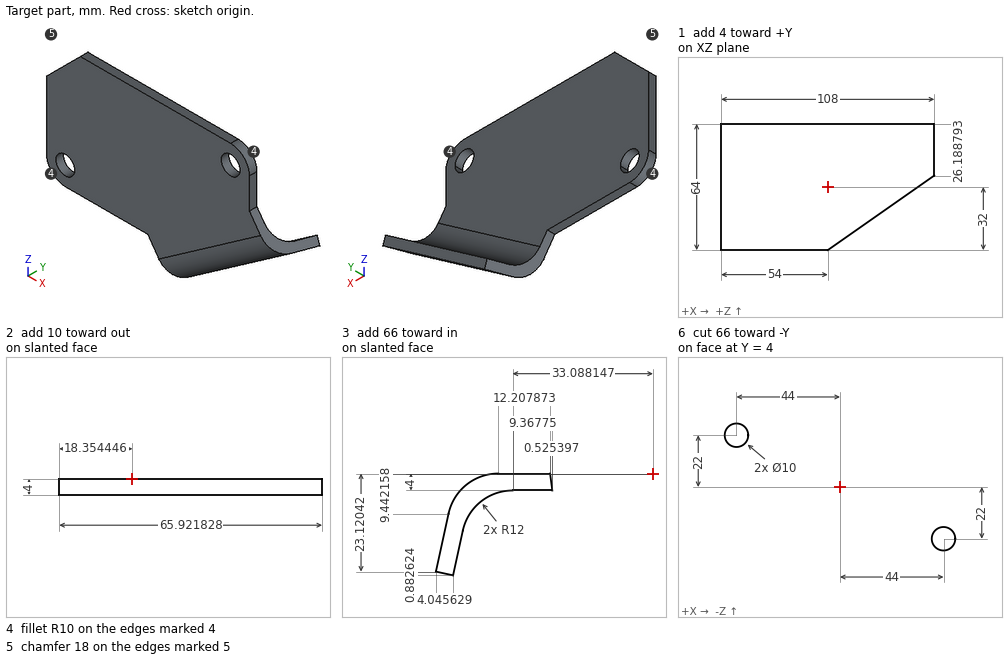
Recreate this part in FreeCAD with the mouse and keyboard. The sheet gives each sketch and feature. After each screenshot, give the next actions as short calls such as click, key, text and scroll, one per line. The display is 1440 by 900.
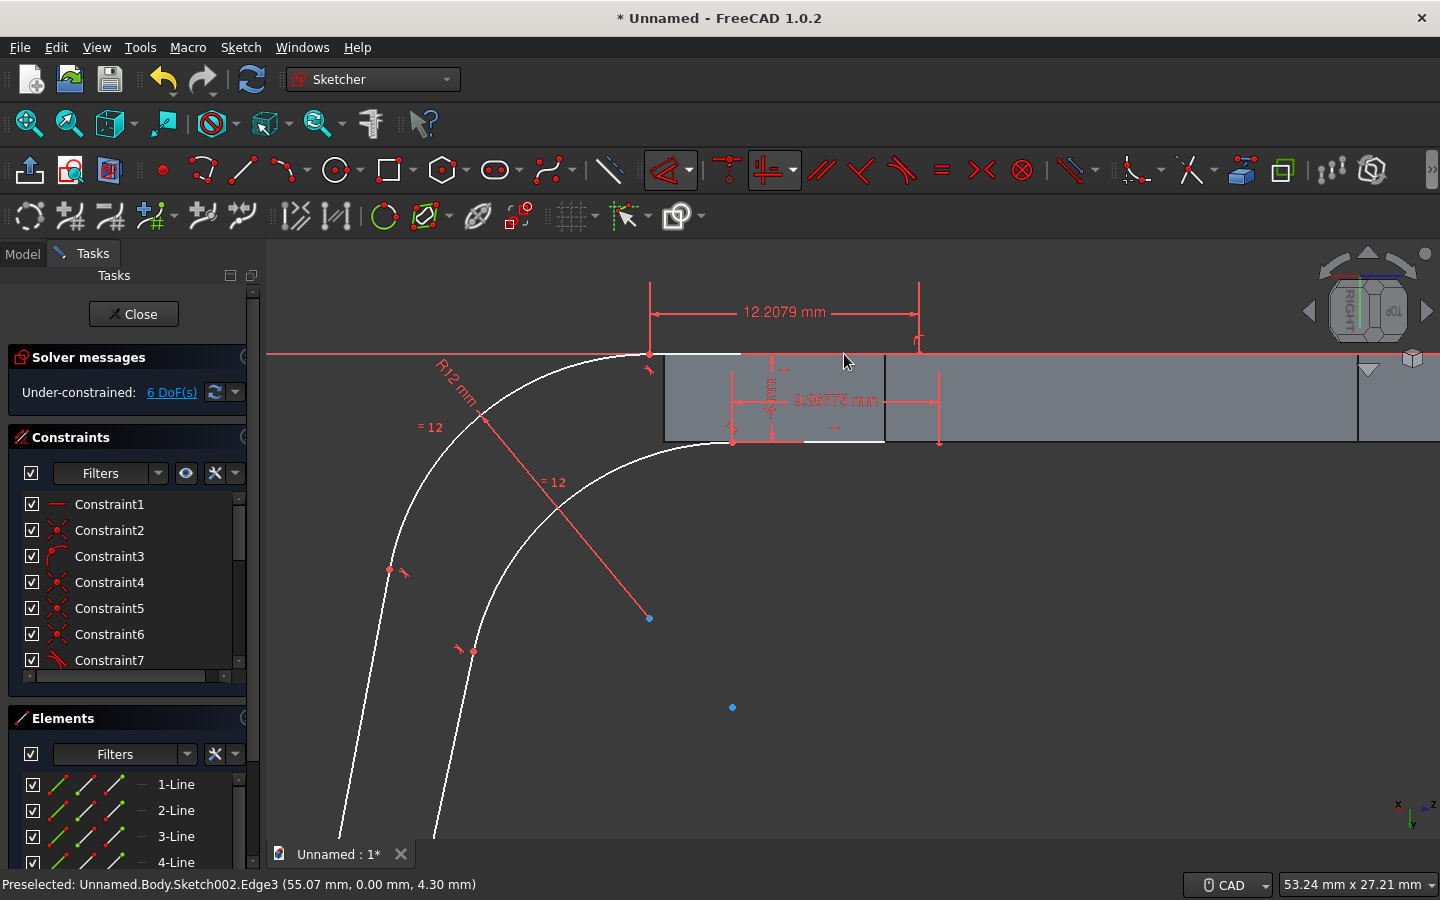
click(390, 570)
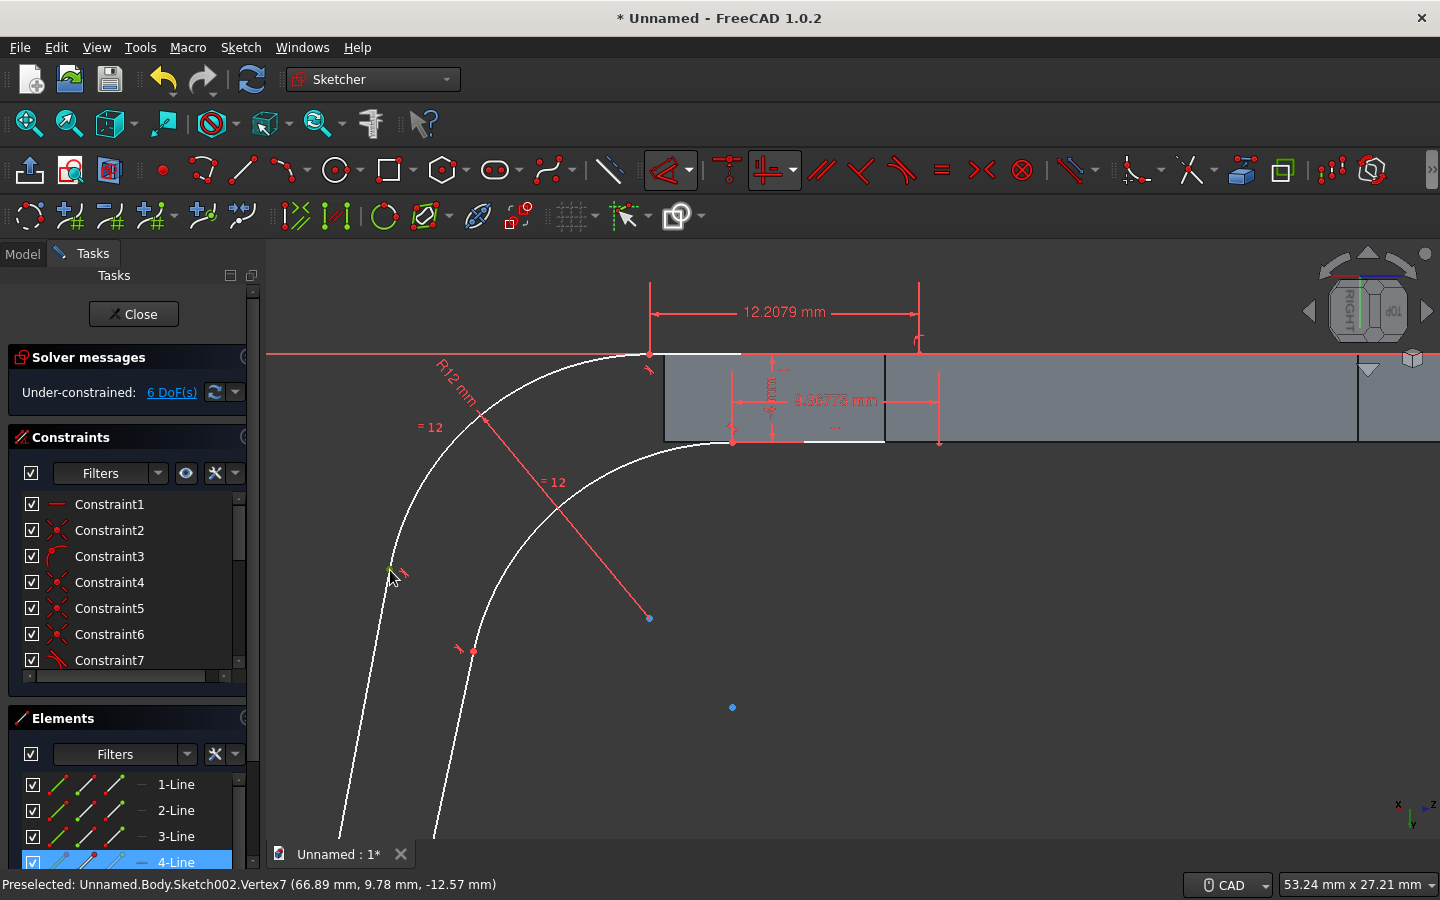
key(i)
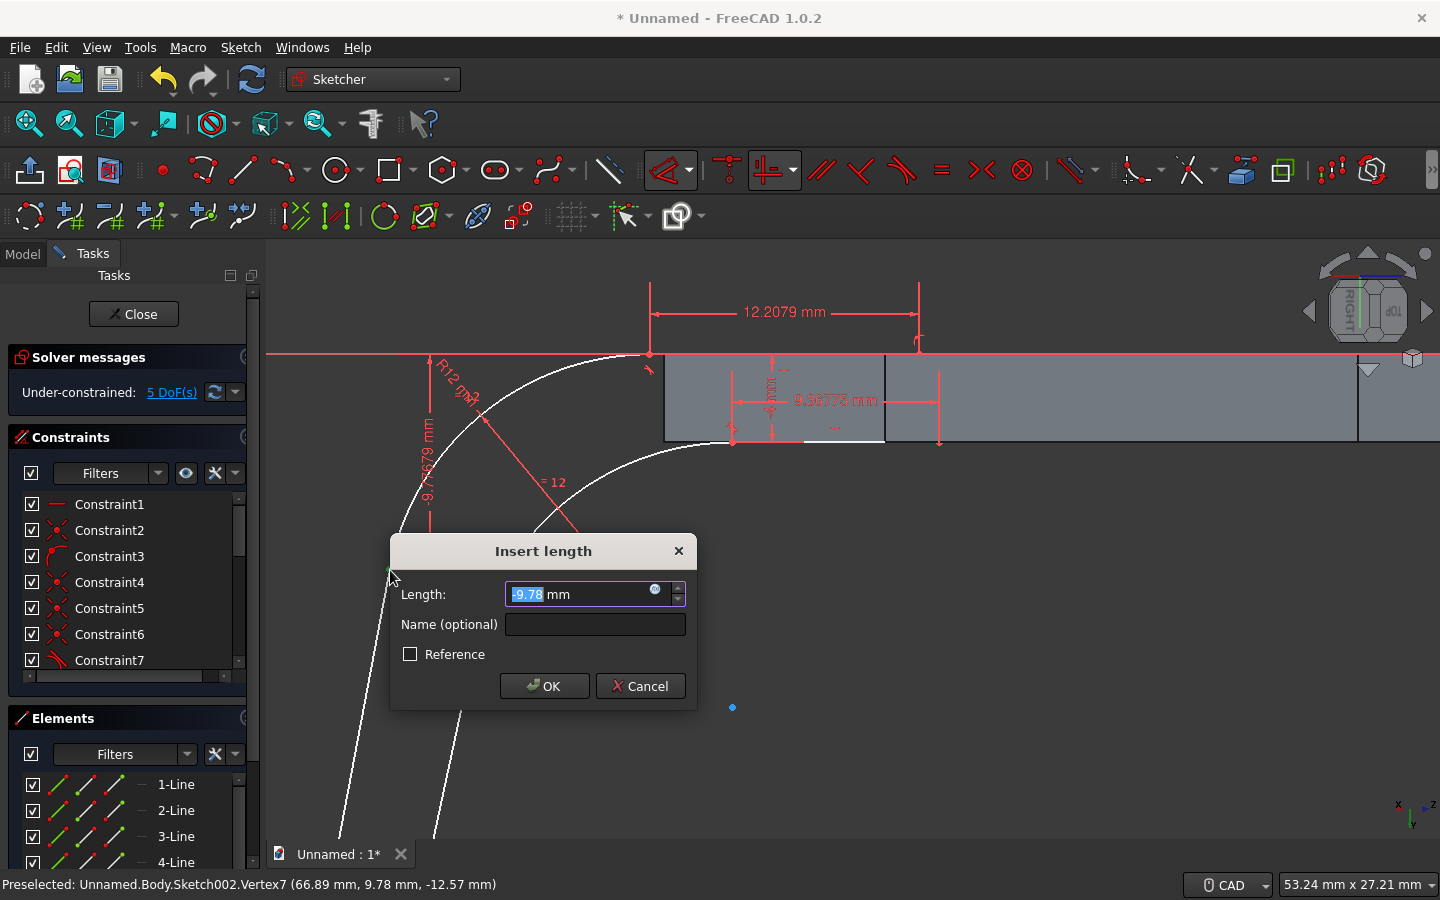
text(-9.442158)
key(Return)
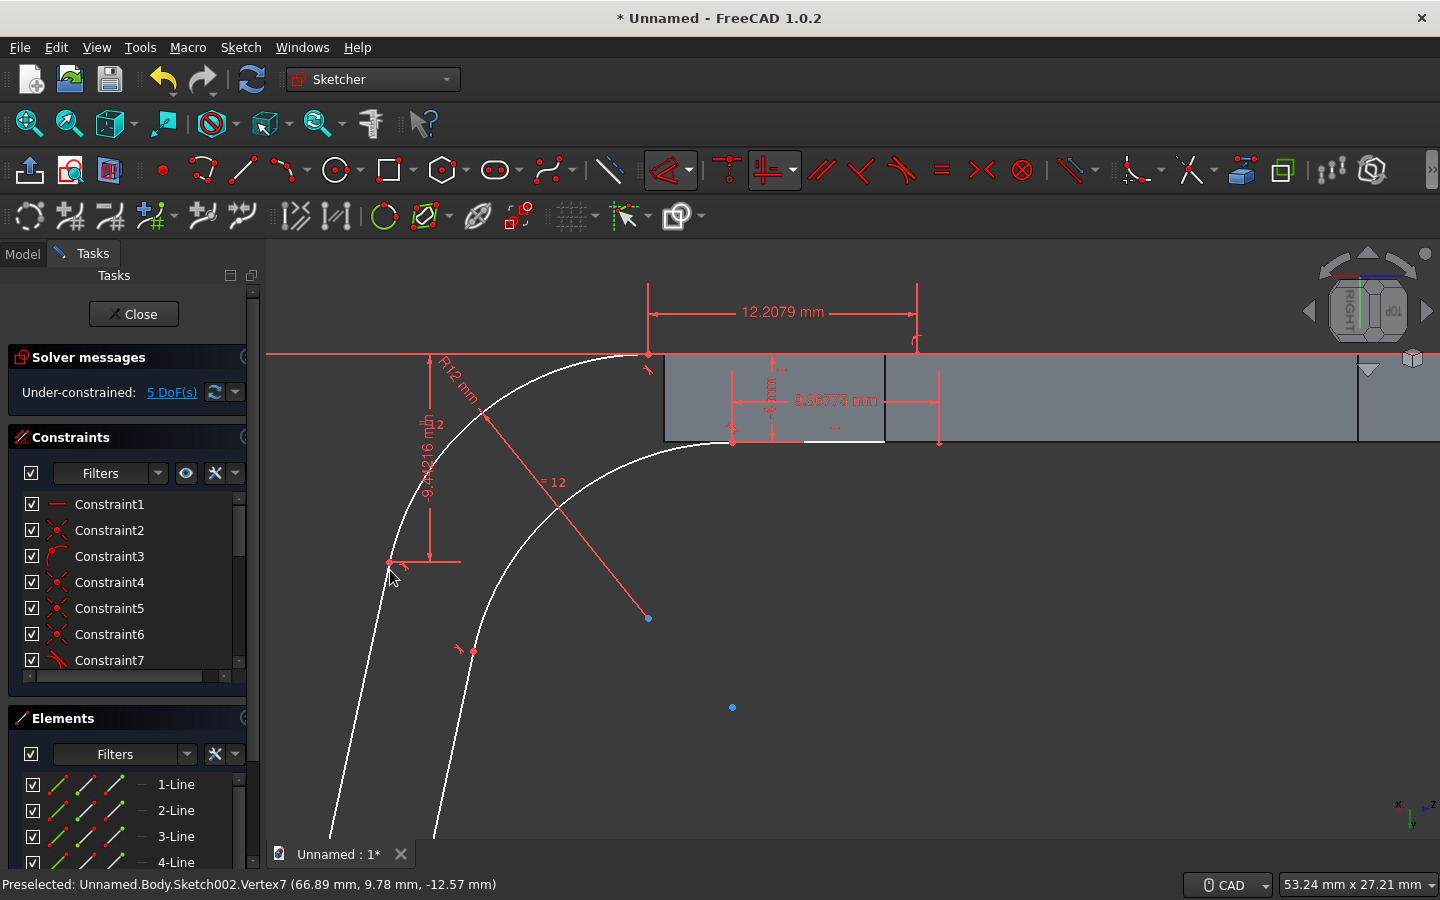
scroll(552, 376, down, 2)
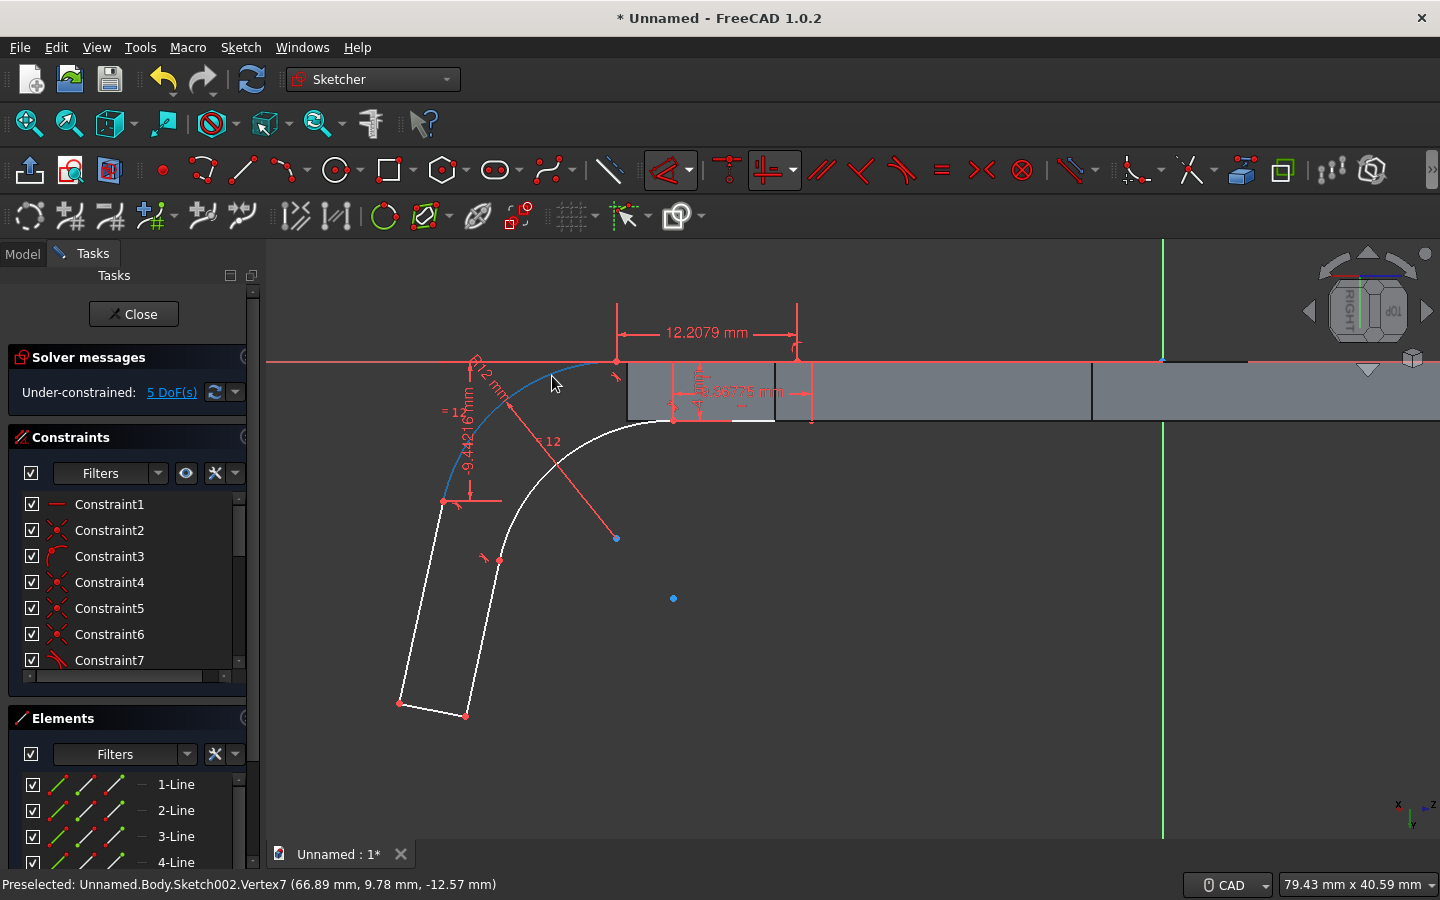
click(399, 704)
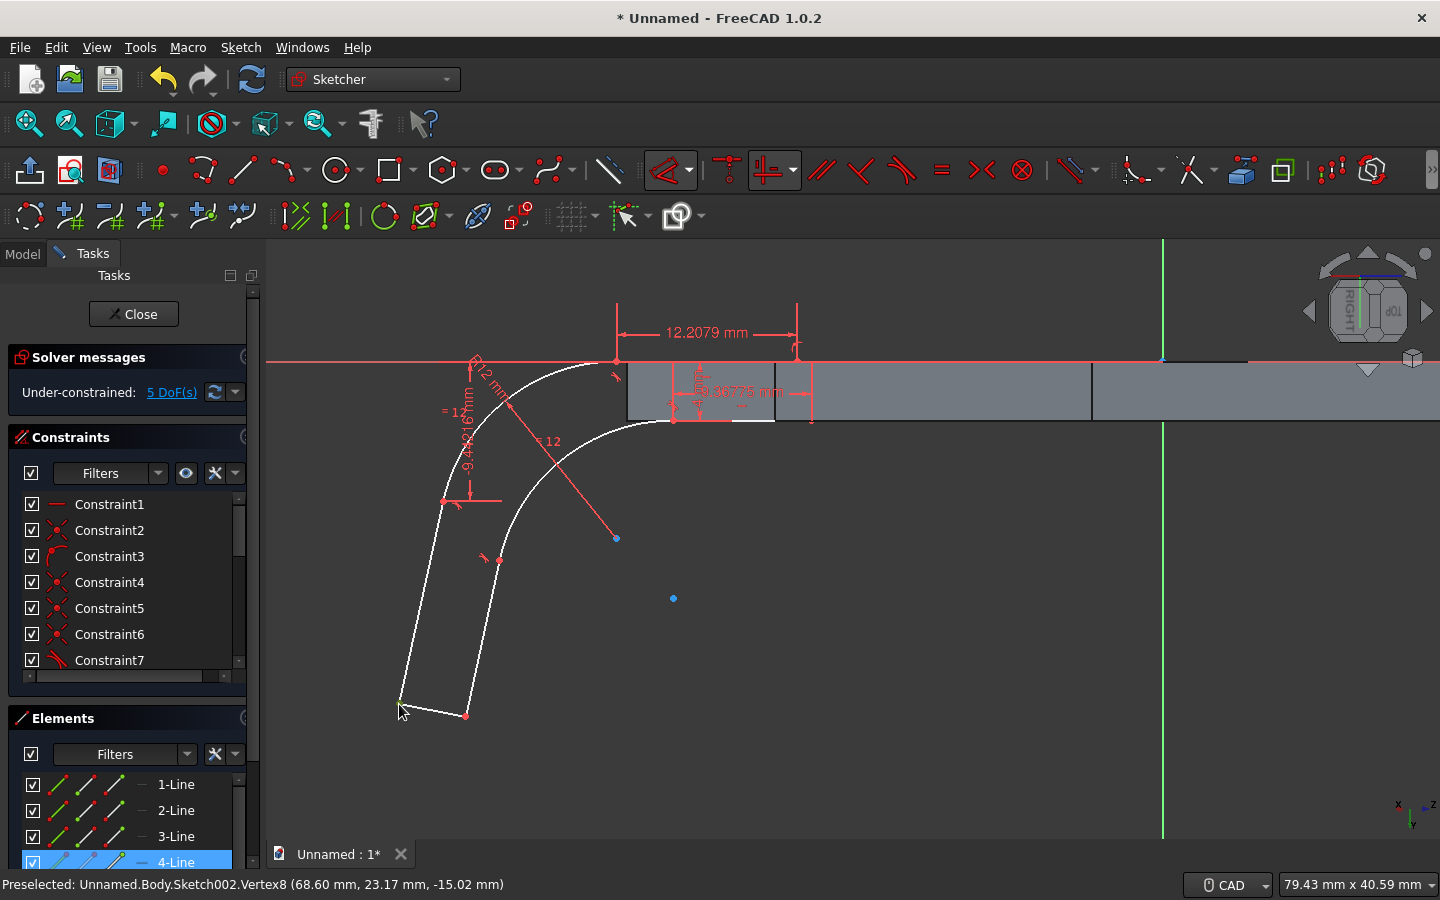
key(i)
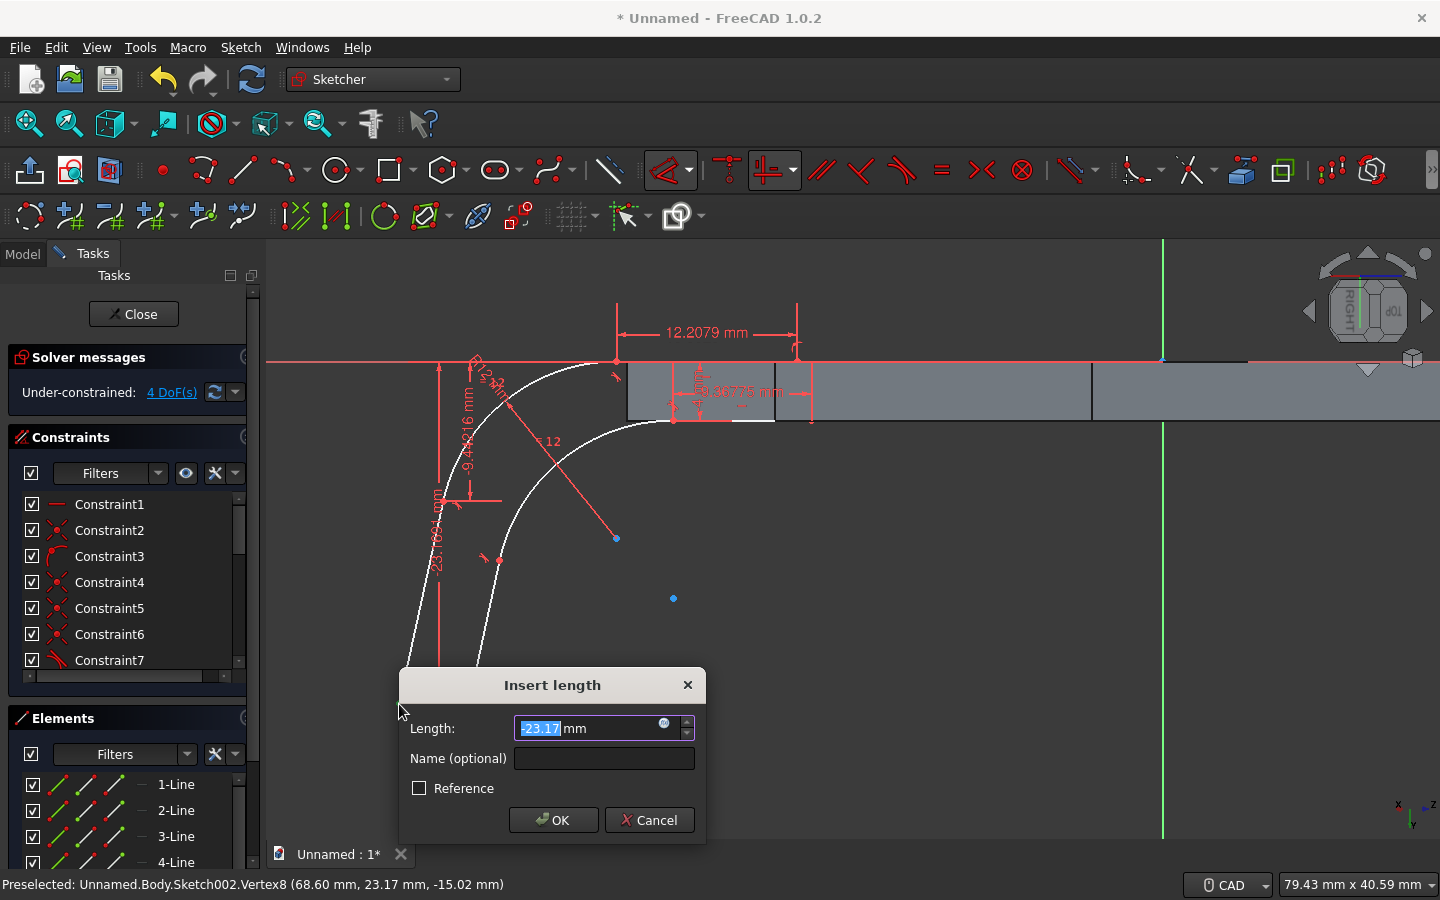
text(-23.12042)
key(Return)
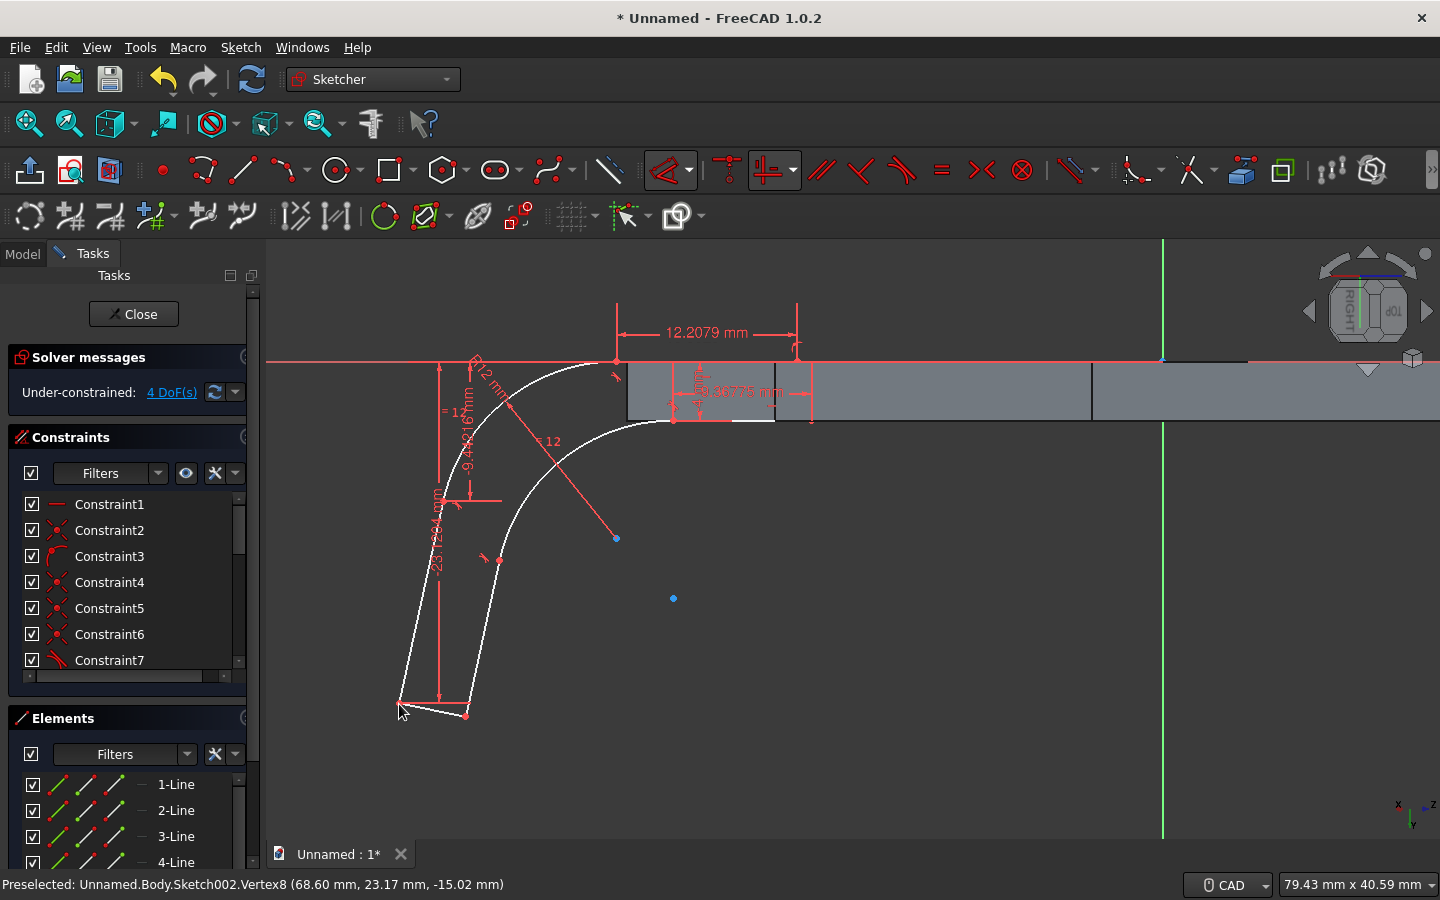
scroll(807, 403, up, 9)